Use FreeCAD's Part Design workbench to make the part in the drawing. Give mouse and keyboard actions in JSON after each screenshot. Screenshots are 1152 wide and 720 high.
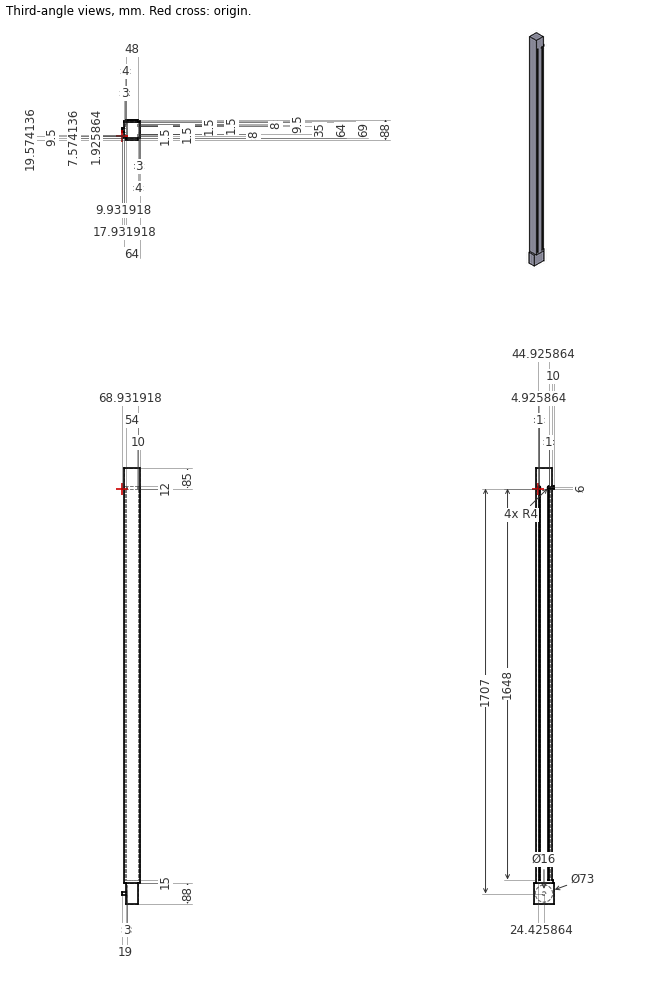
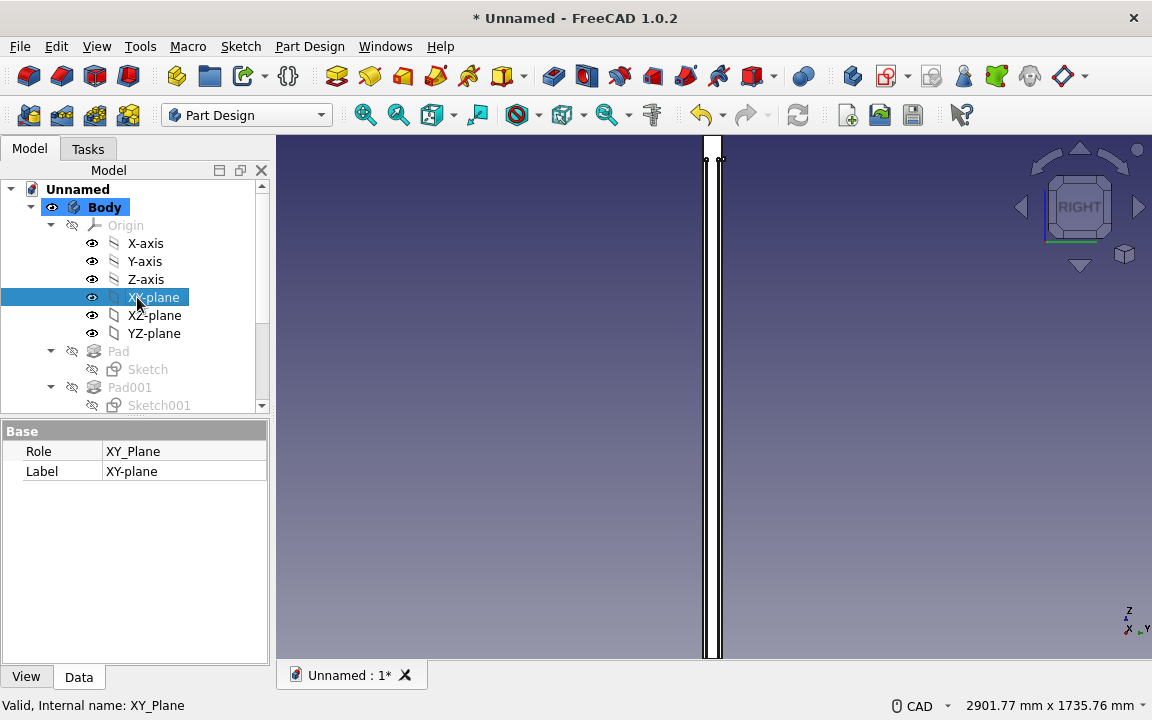
{"action": "left_click", "coordinate": [1062, 76]}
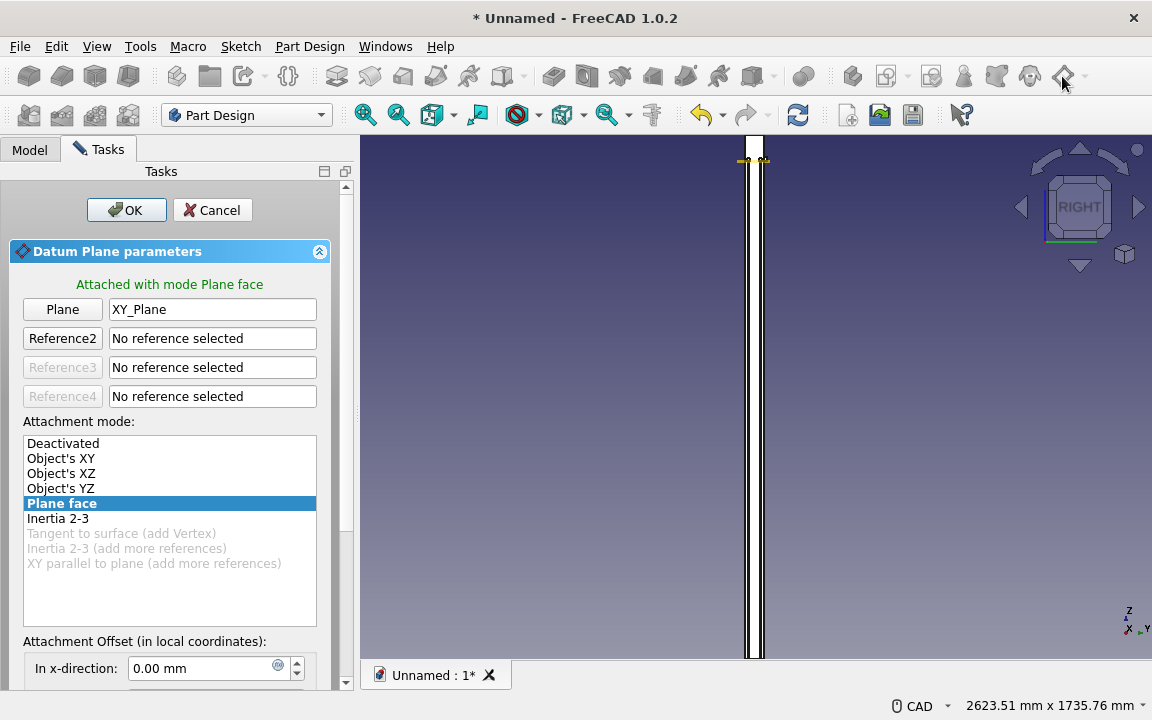
{"action": "scroll", "coordinate": [346, 436], "scroll_direction": "down", "scroll_amount": 2}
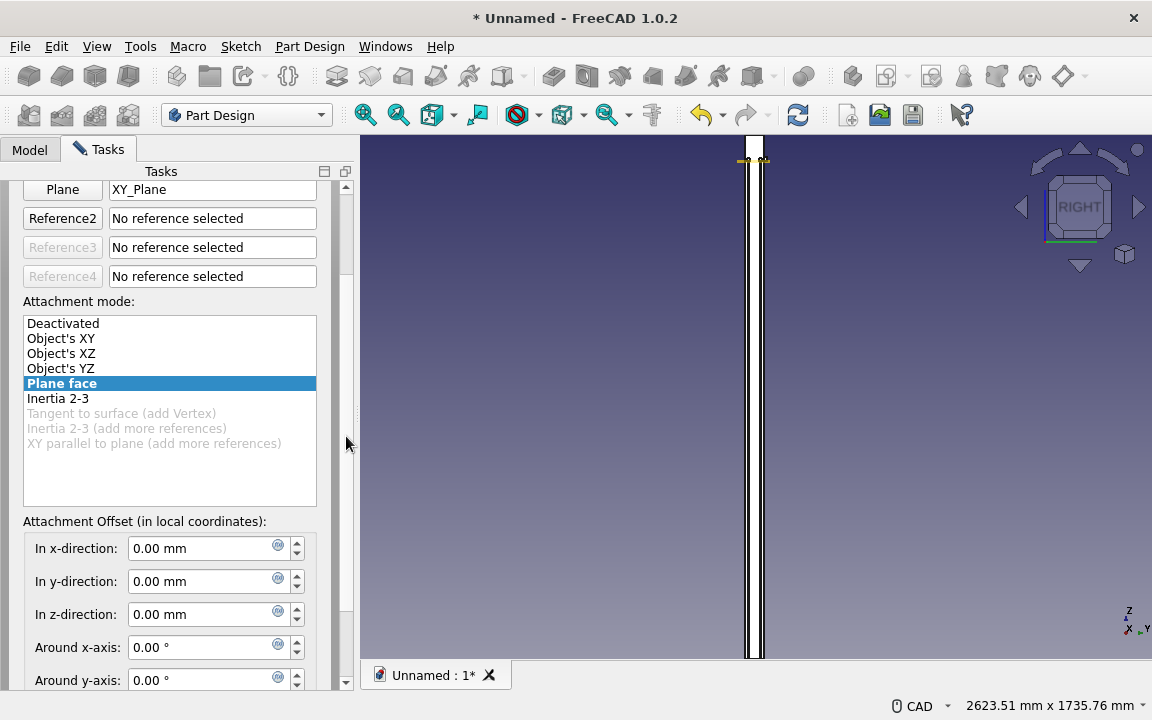
{"action": "triple_click", "coordinate": [210, 614]}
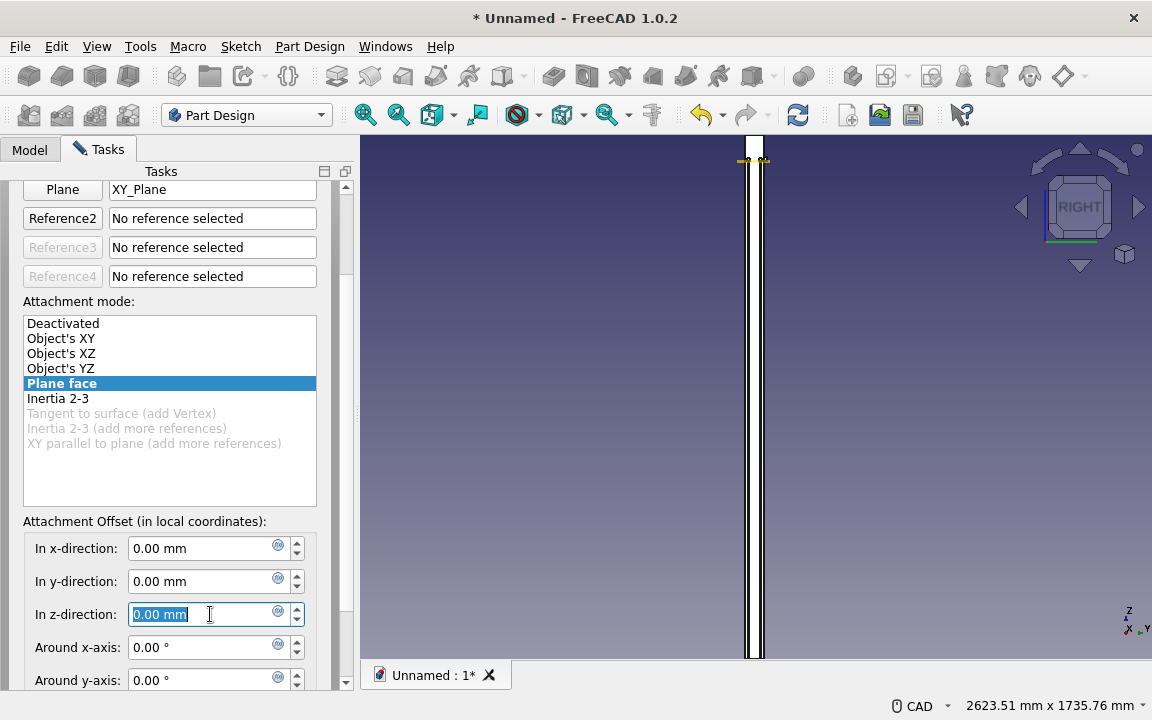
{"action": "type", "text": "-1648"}
{"action": "key", "text": "Tab"}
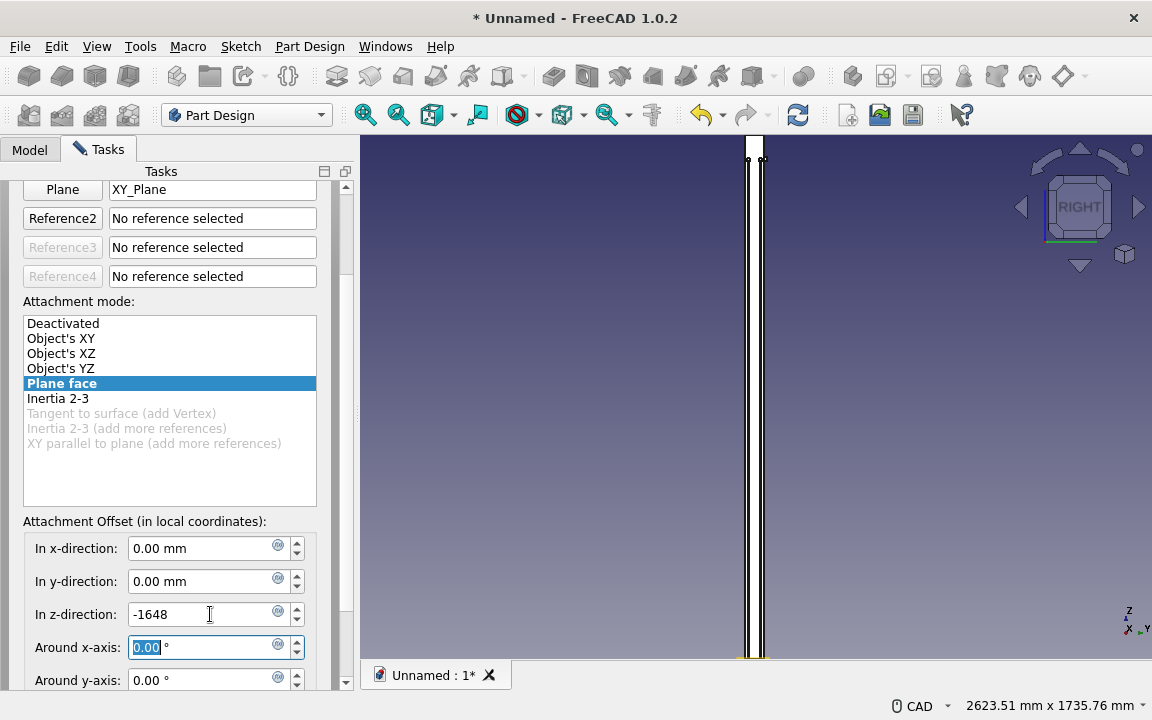
{"action": "scroll", "coordinate": [346, 436], "scroll_direction": "up", "scroll_amount": 3}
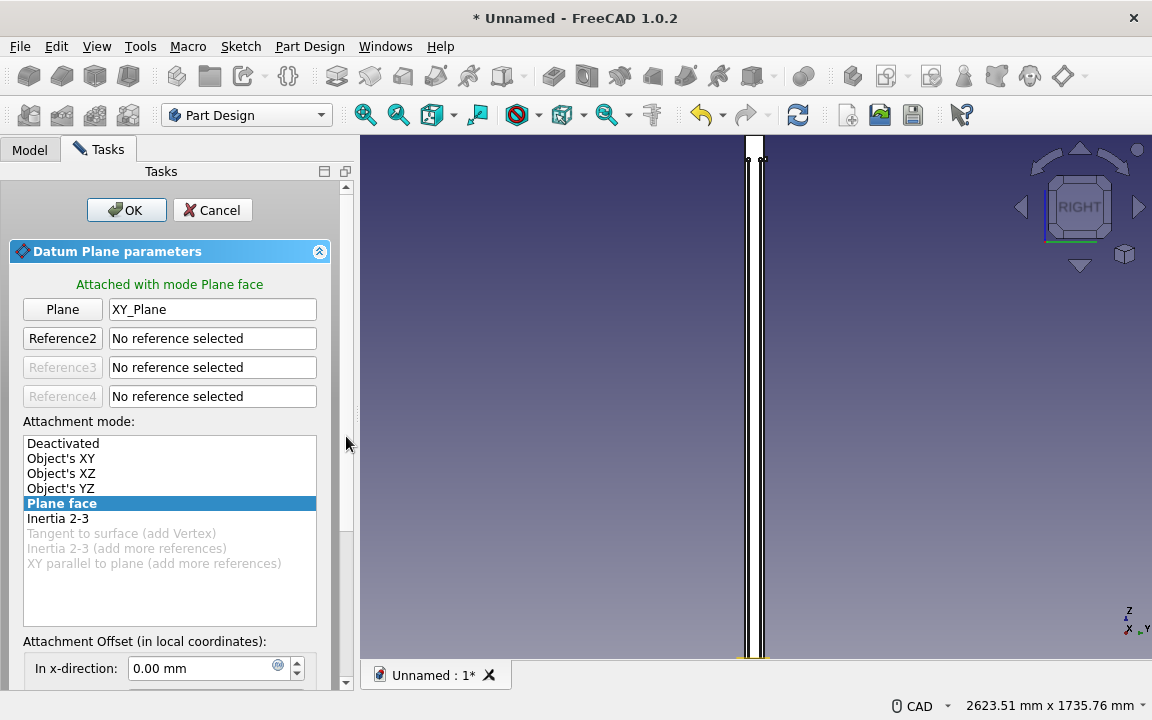
{"action": "left_click", "coordinate": [127, 210]}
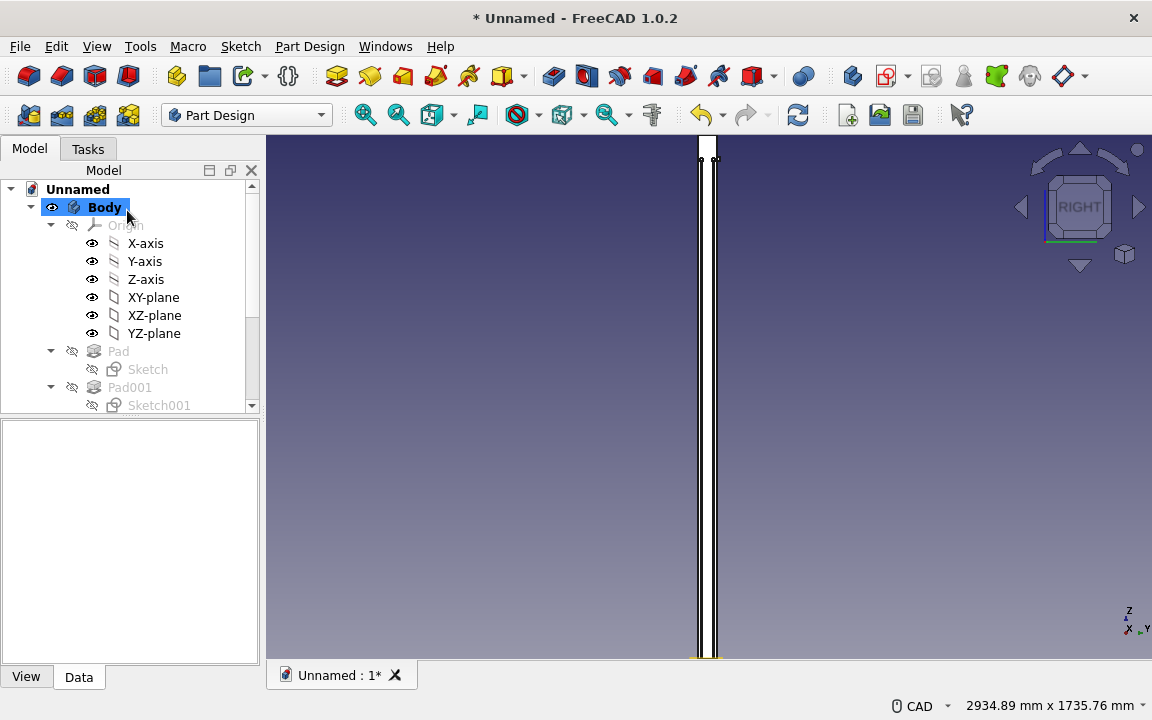
{"action": "scroll", "coordinate": [101, 293], "scroll_direction": "down", "scroll_amount": 3}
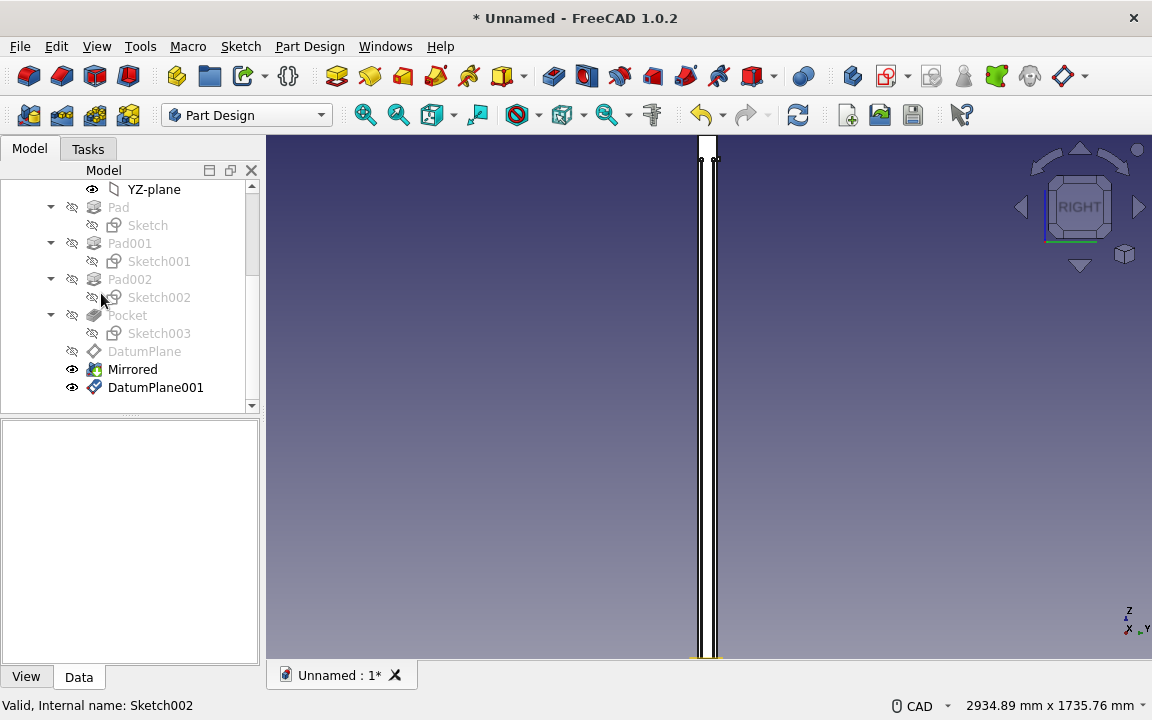
{"action": "left_click", "coordinate": [117, 387]}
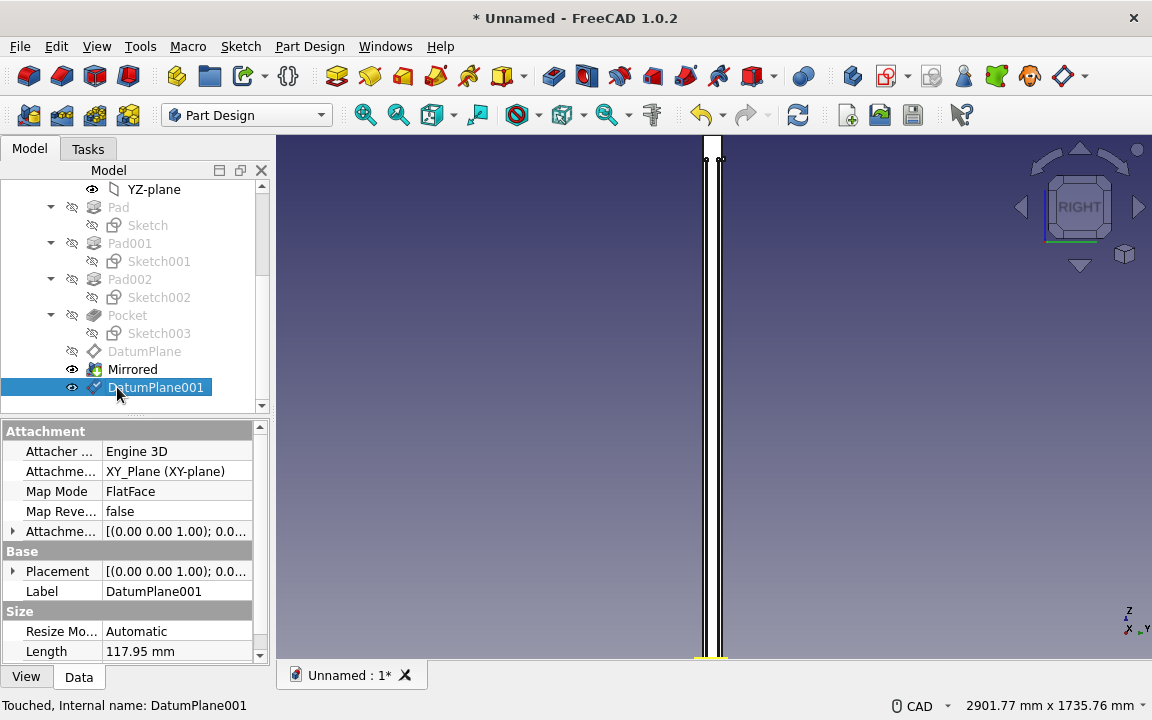
{"action": "left_click", "coordinate": [886, 76]}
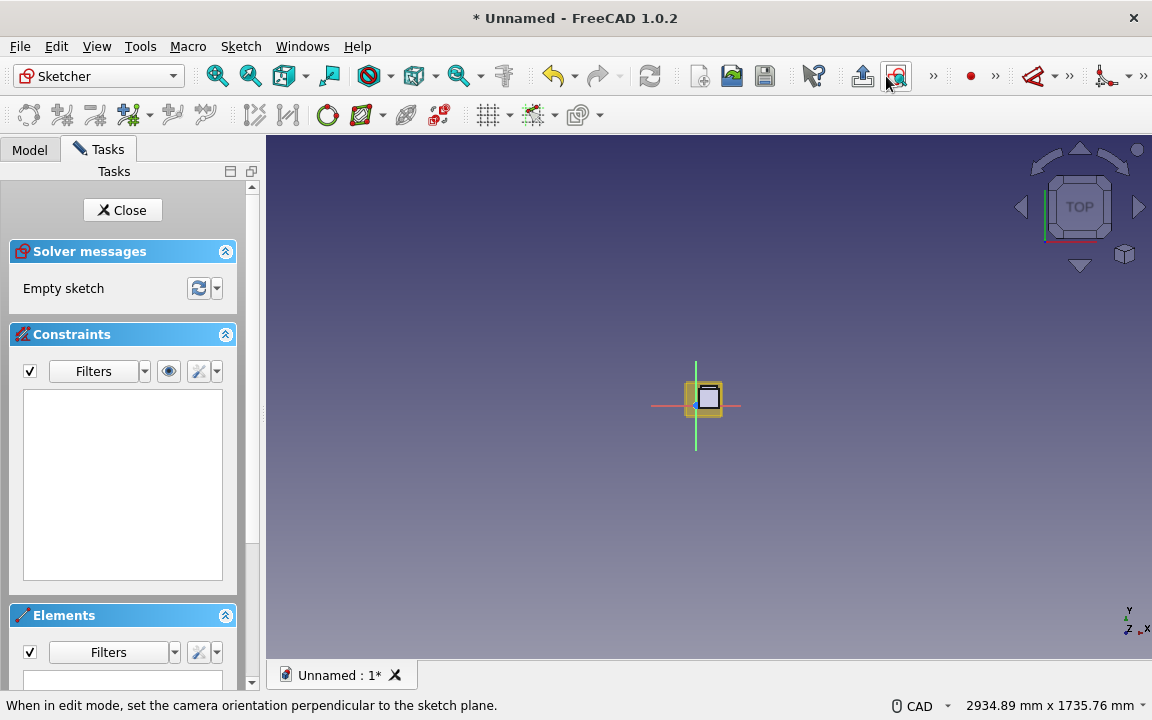
{"action": "key", "text": "q s"}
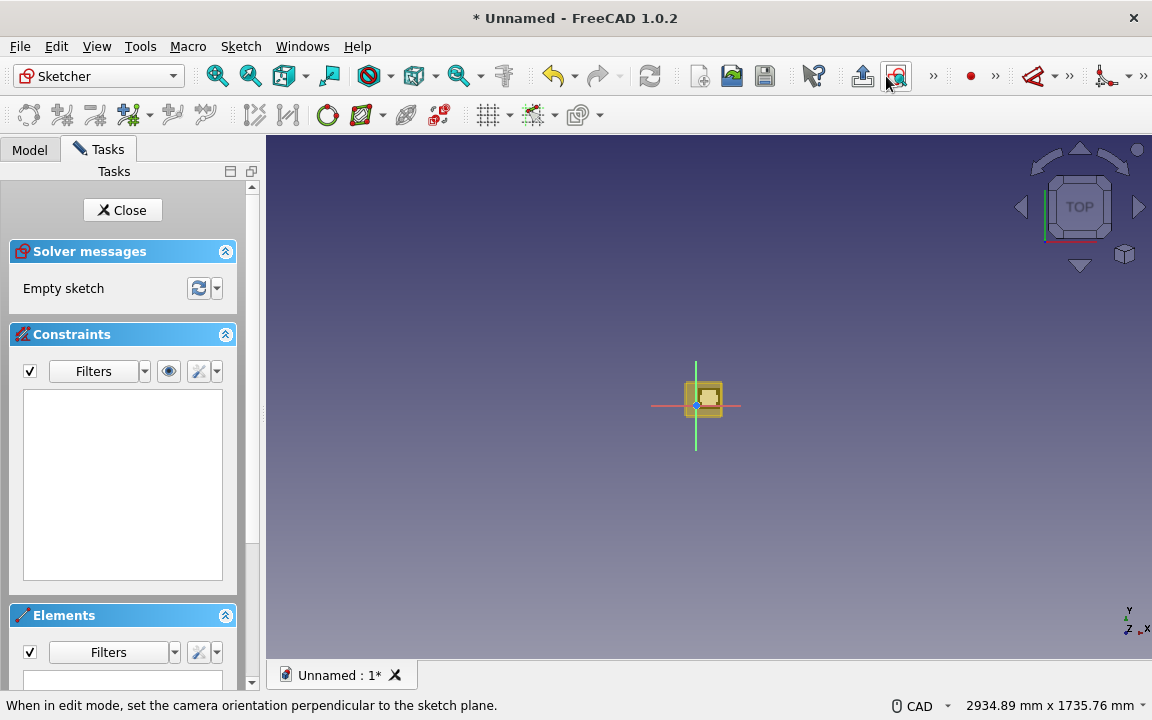
{"action": "scroll", "coordinate": [712, 398], "scroll_direction": "up", "scroll_amount": 14}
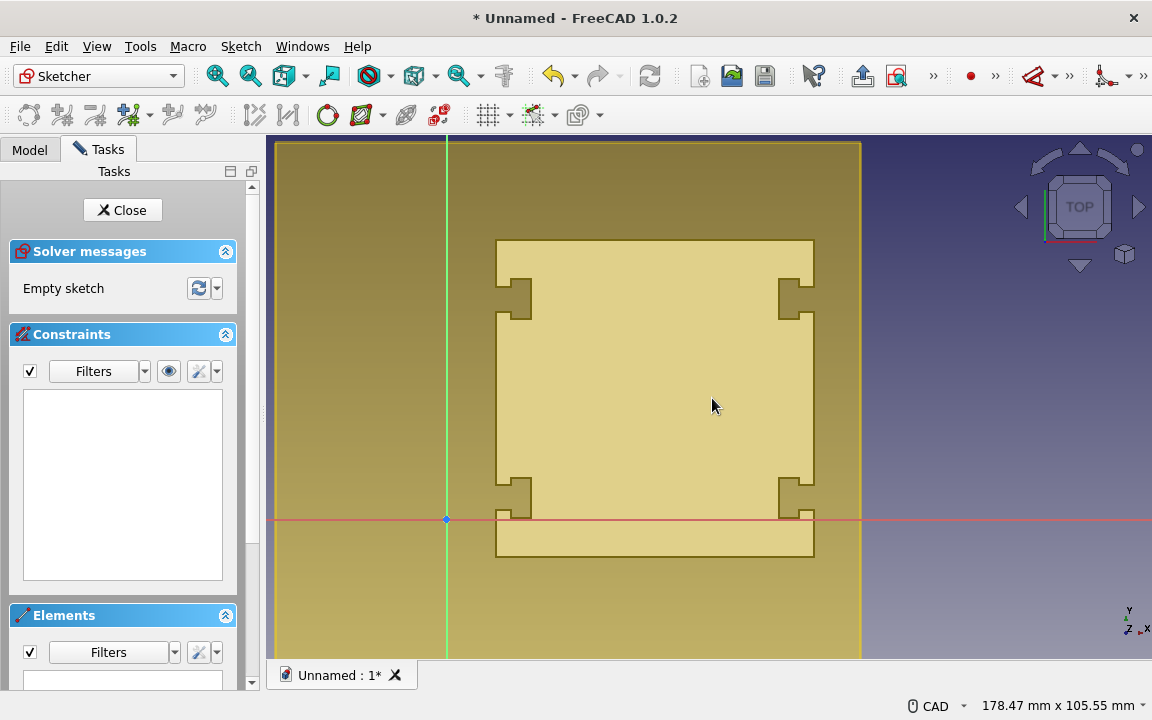
{"action": "key", "text": "g r"}